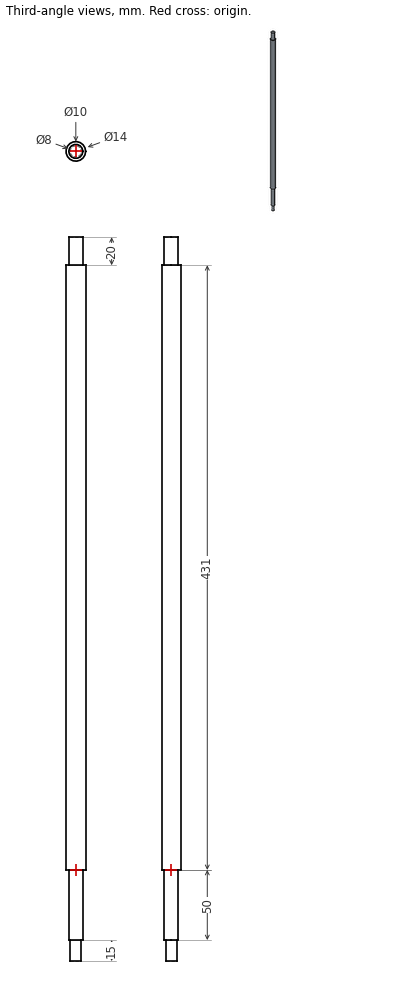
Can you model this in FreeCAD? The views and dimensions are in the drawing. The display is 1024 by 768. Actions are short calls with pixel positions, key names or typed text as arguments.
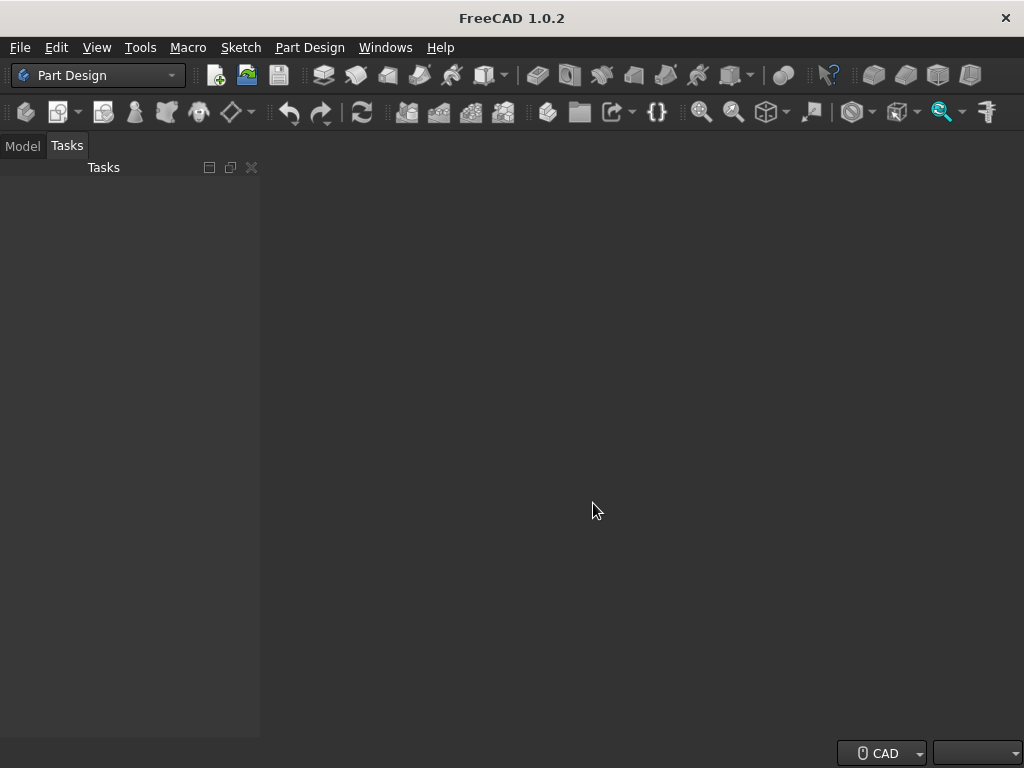
click(216, 76)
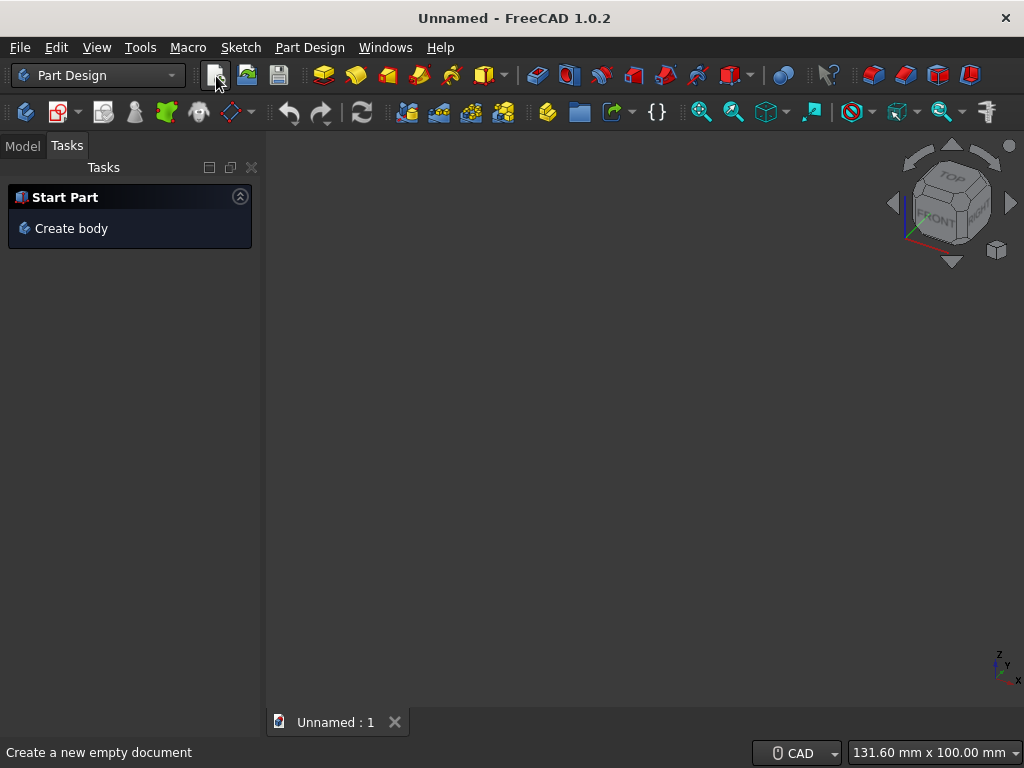
click(58, 112)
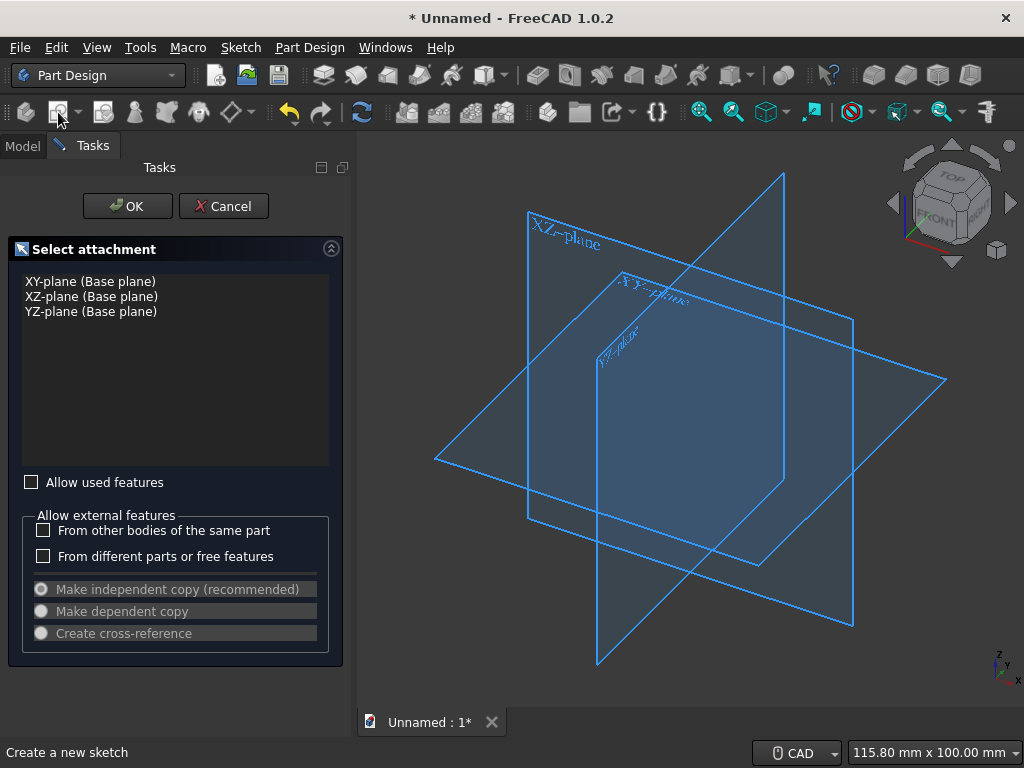
click(82, 282)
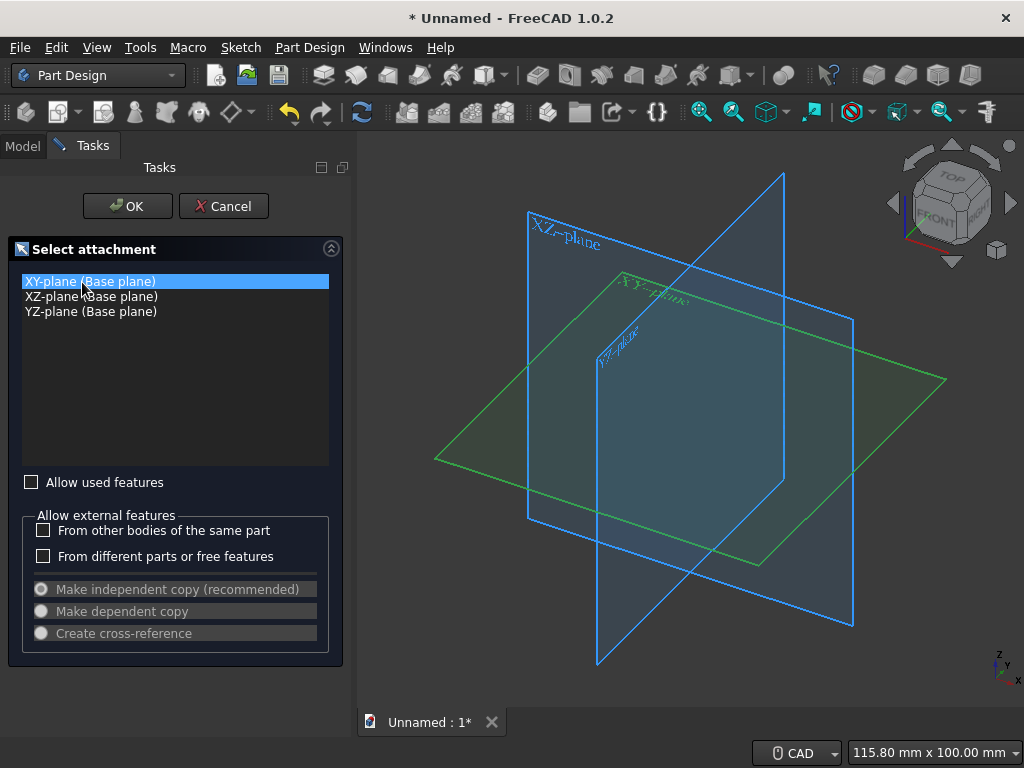
click(128, 206)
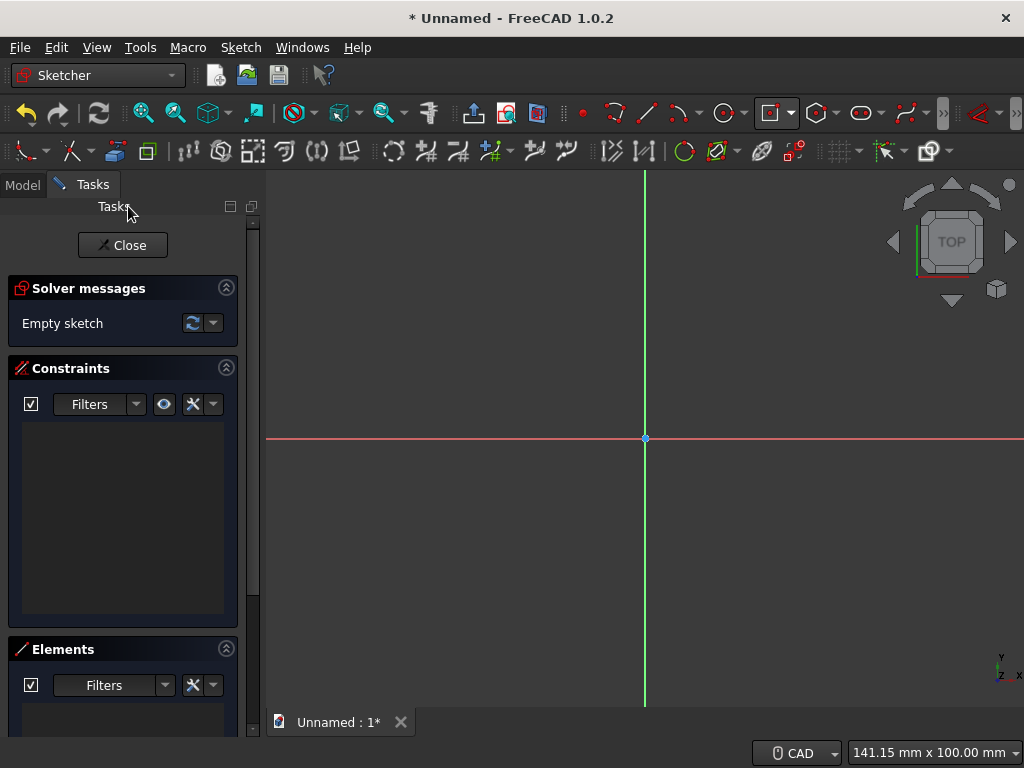
scroll(662, 438, up, 8)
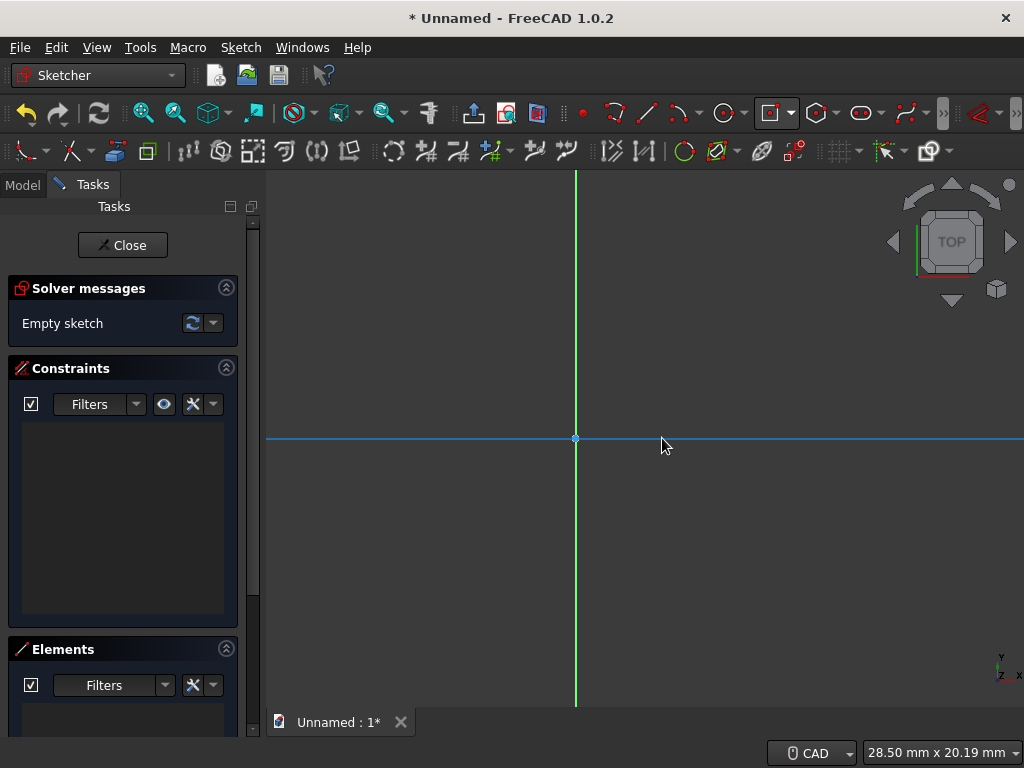
click(724, 114)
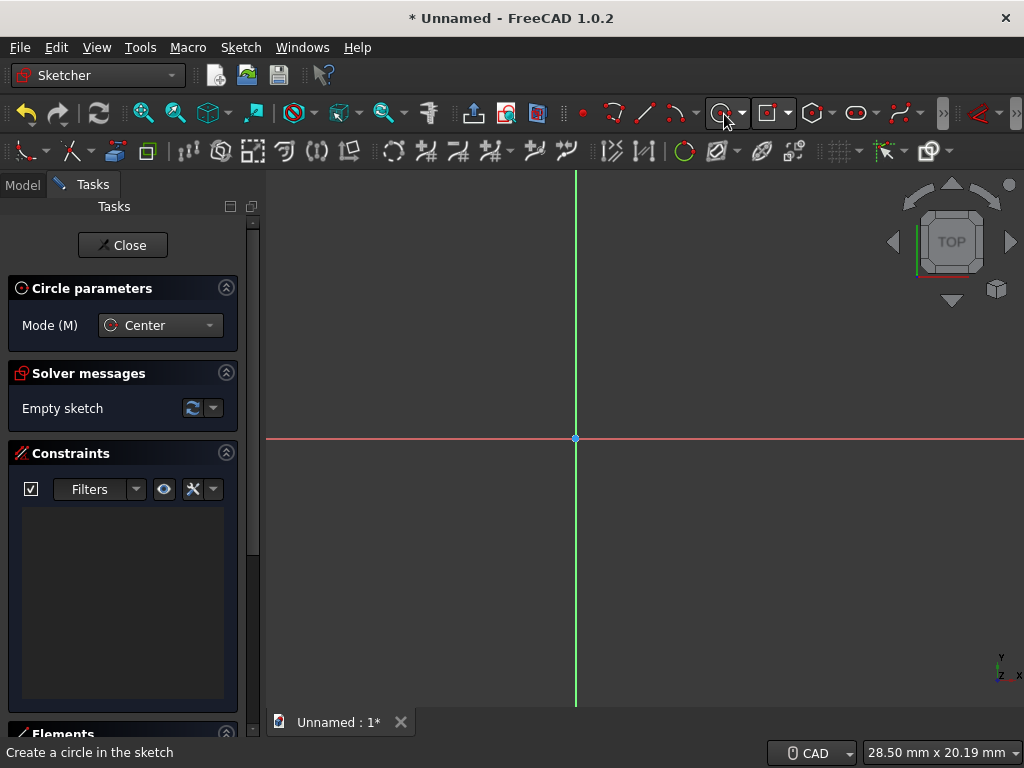
click(576, 438)
move(707, 307)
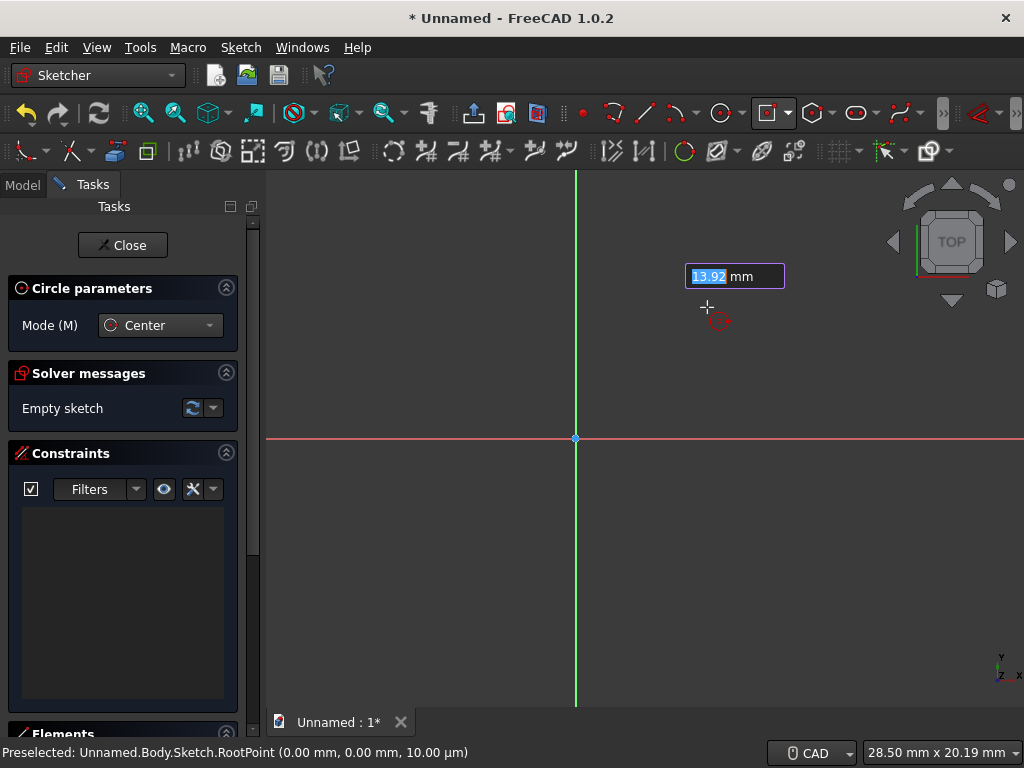
text(14)
key(Return)
key(Escape)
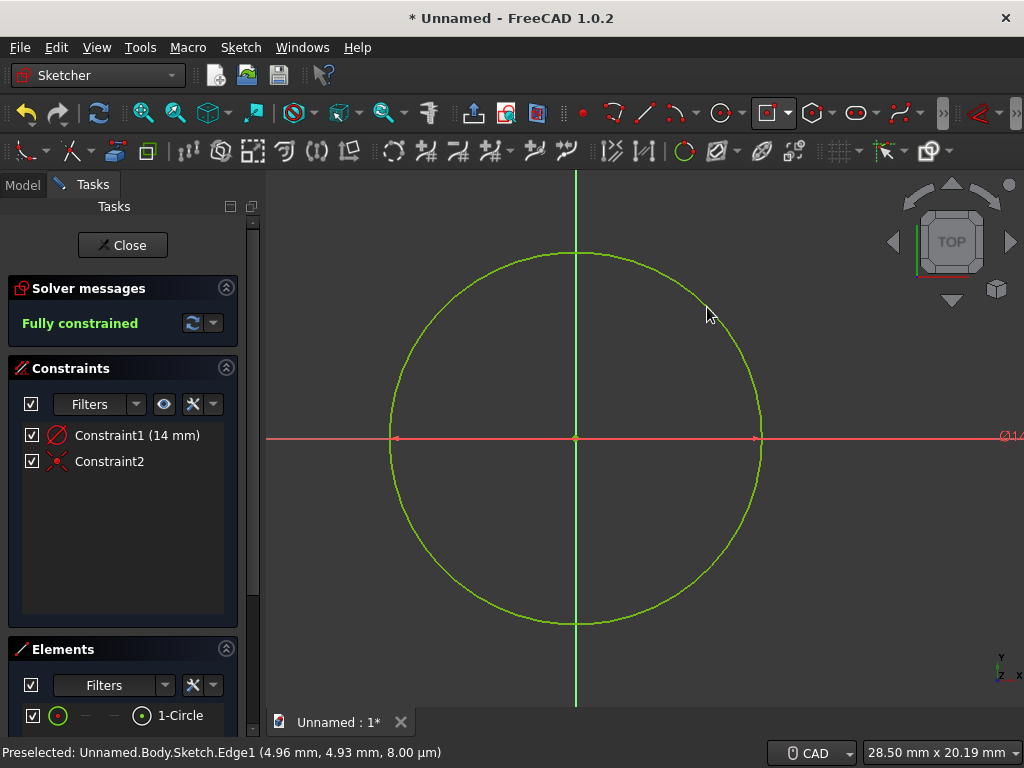
click(123, 245)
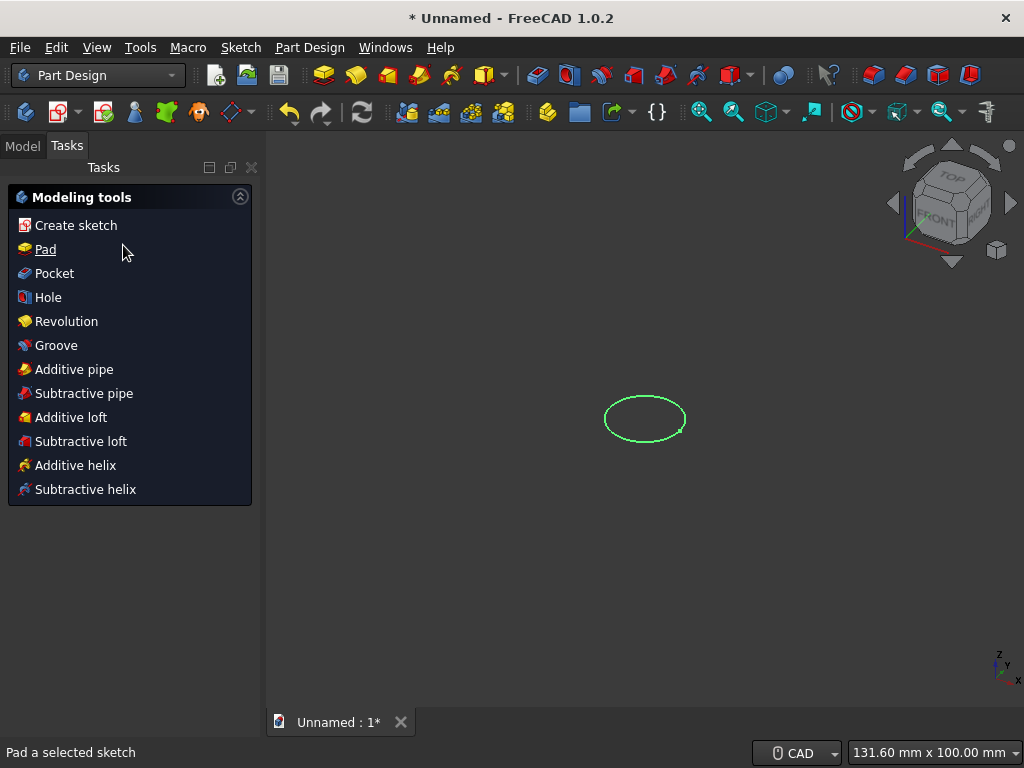
click(324, 76)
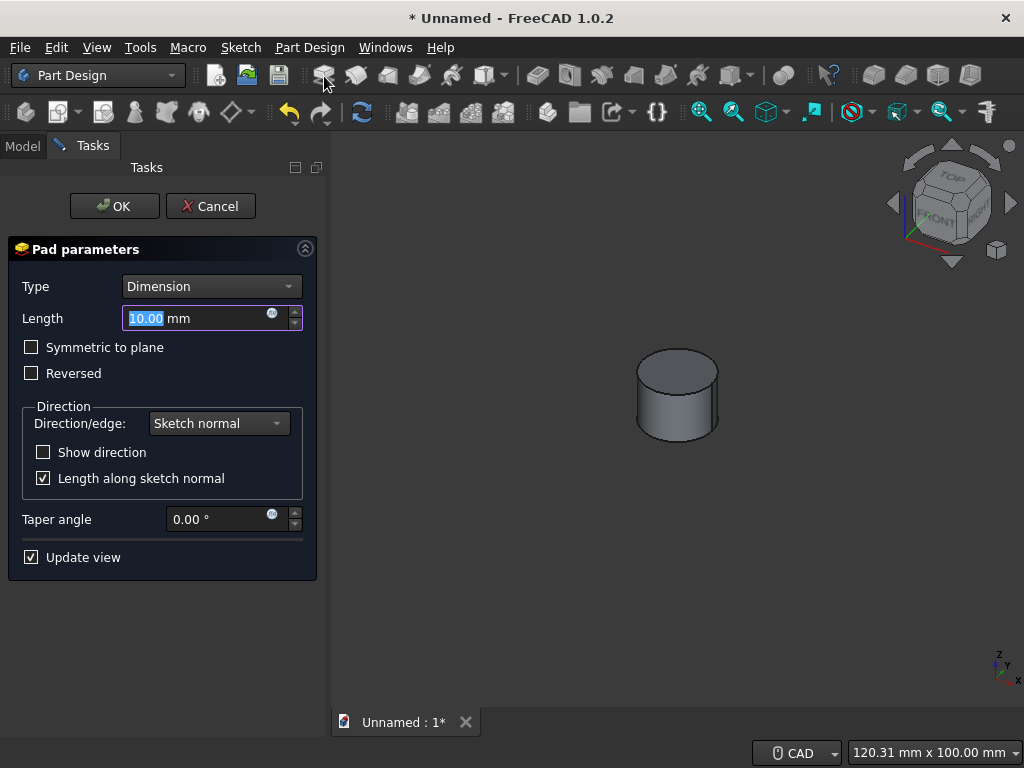
text(431)
key(Tab)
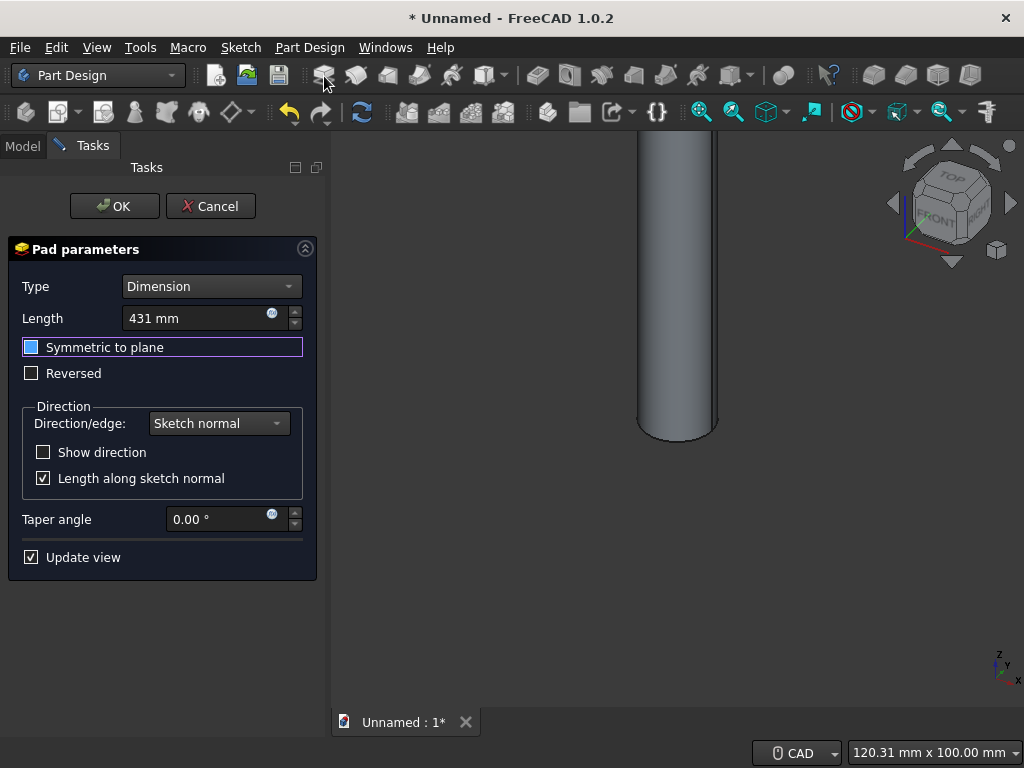
click(115, 206)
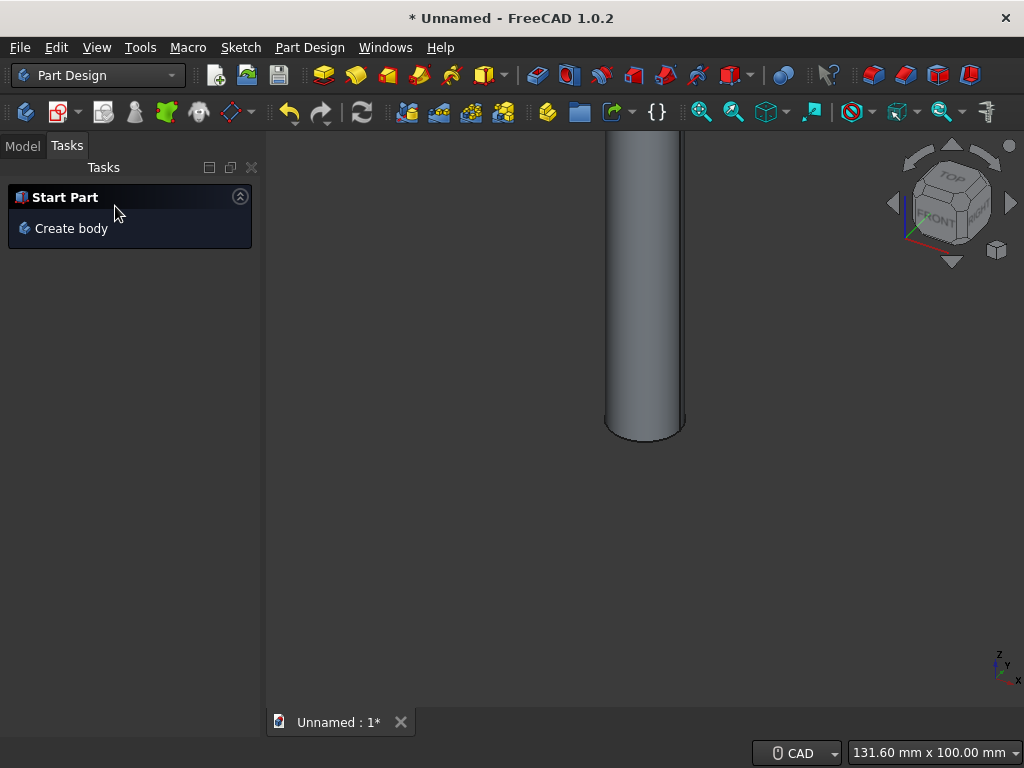
click(702, 112)